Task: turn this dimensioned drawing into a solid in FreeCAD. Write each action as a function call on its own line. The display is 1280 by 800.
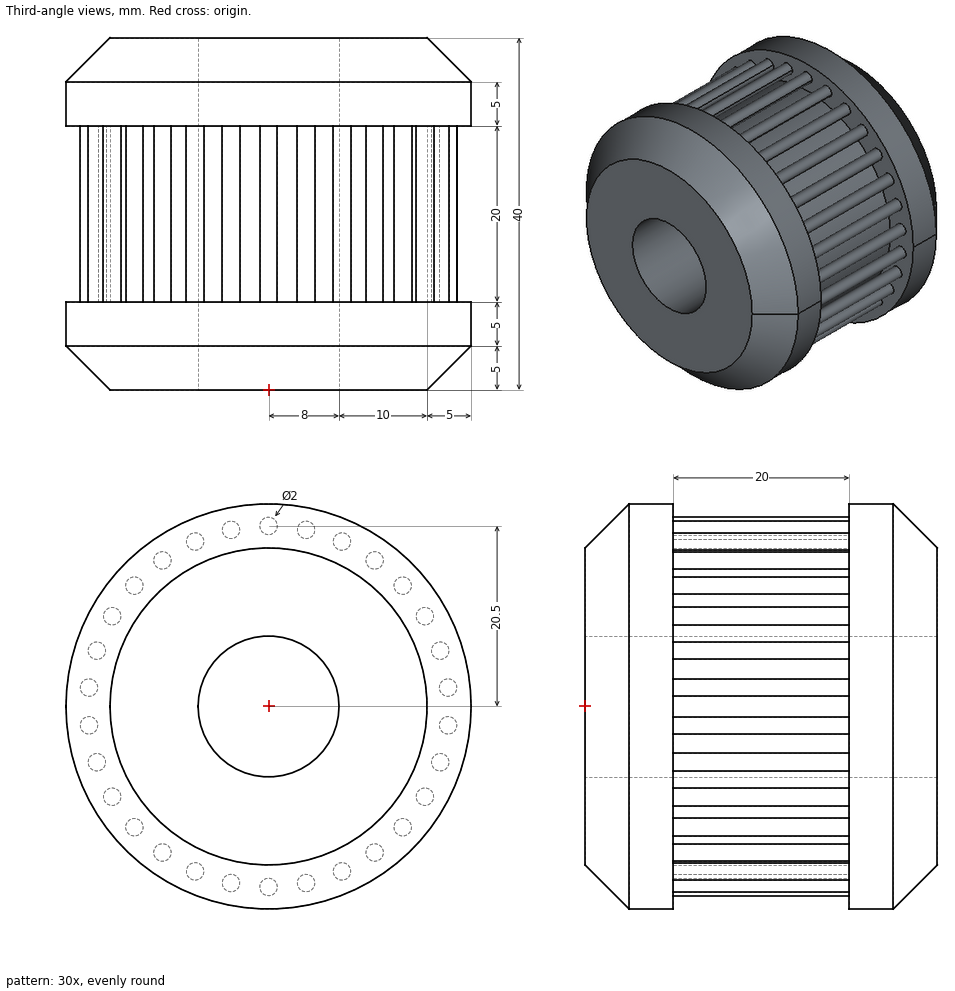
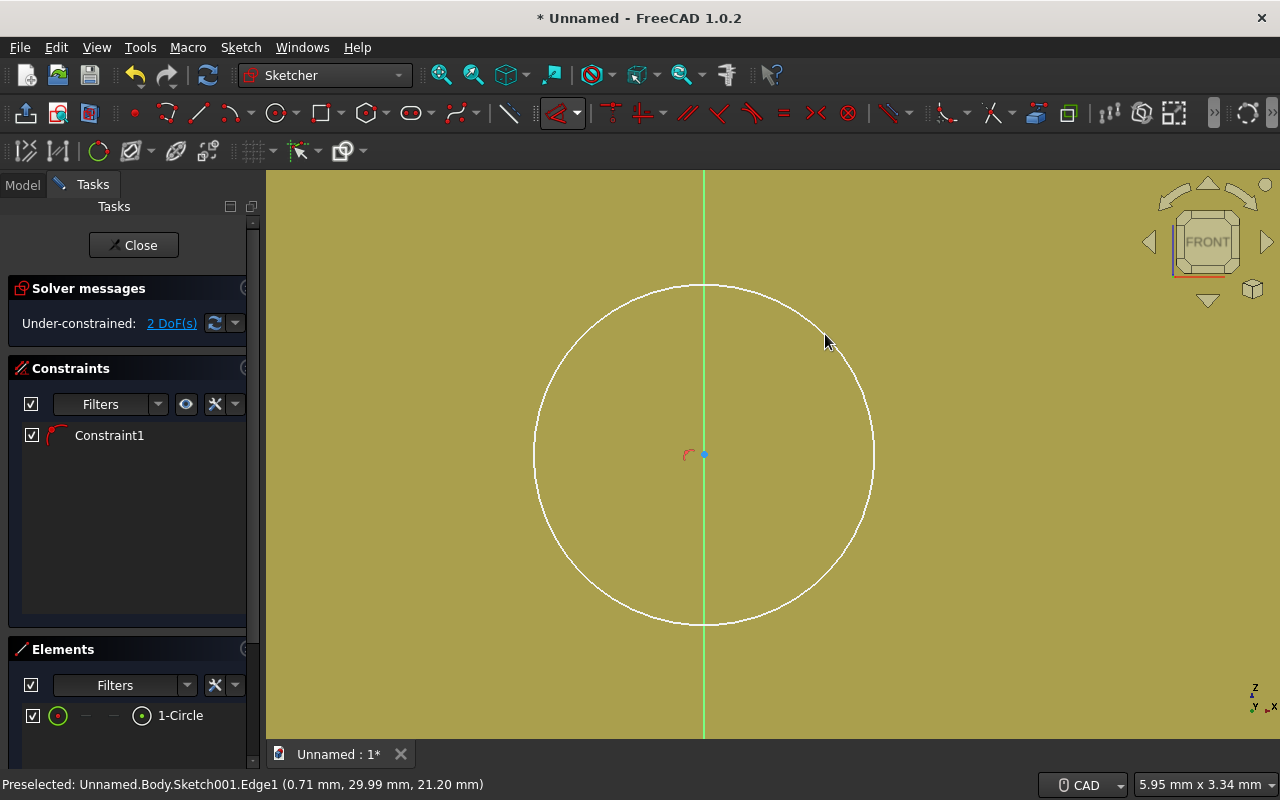
click(824, 334)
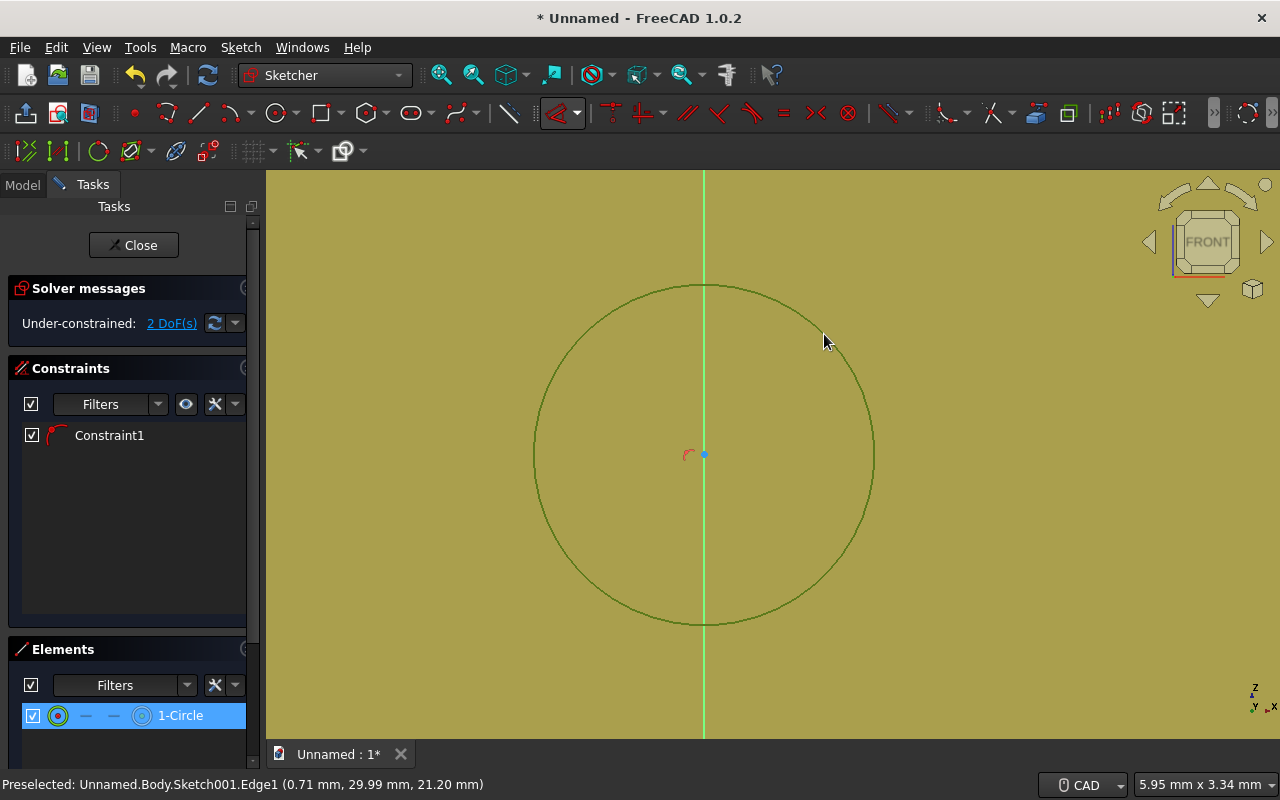
click(580, 114)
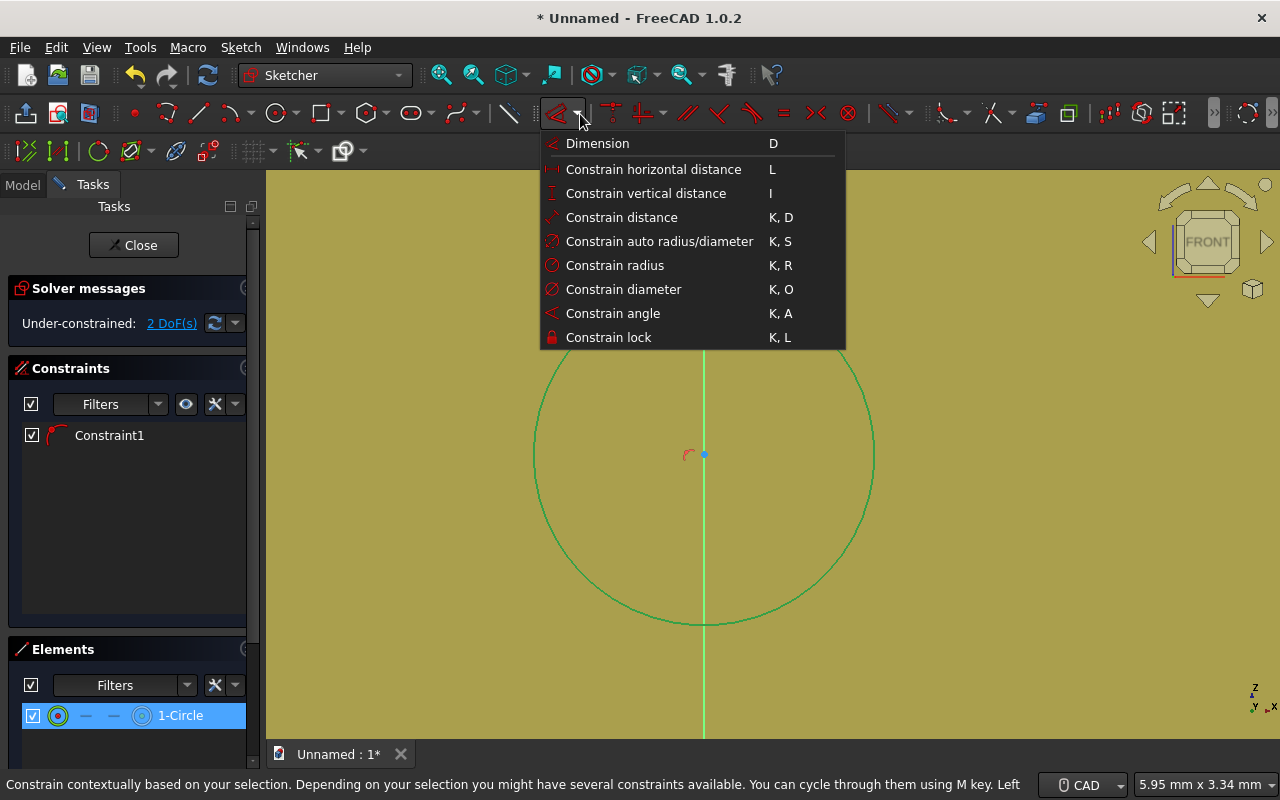
click(693, 289)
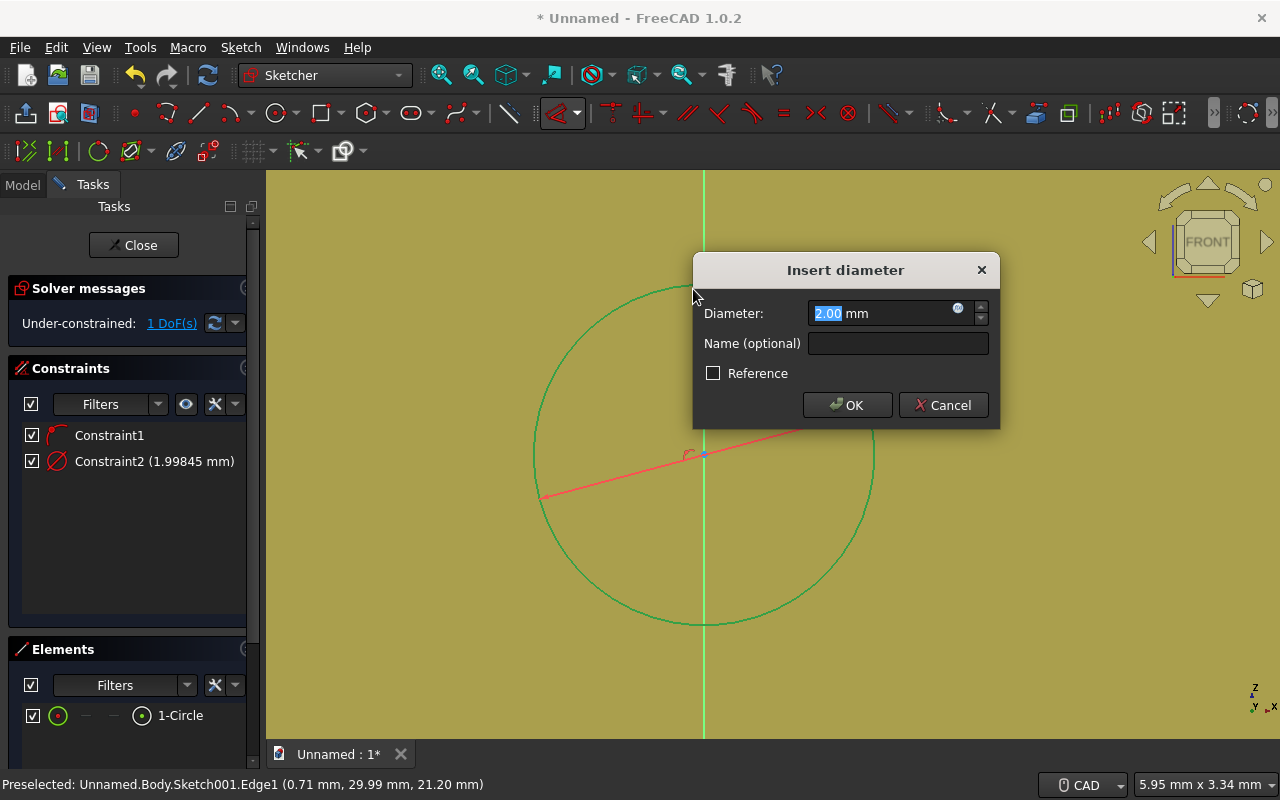
text(2)
key(Return)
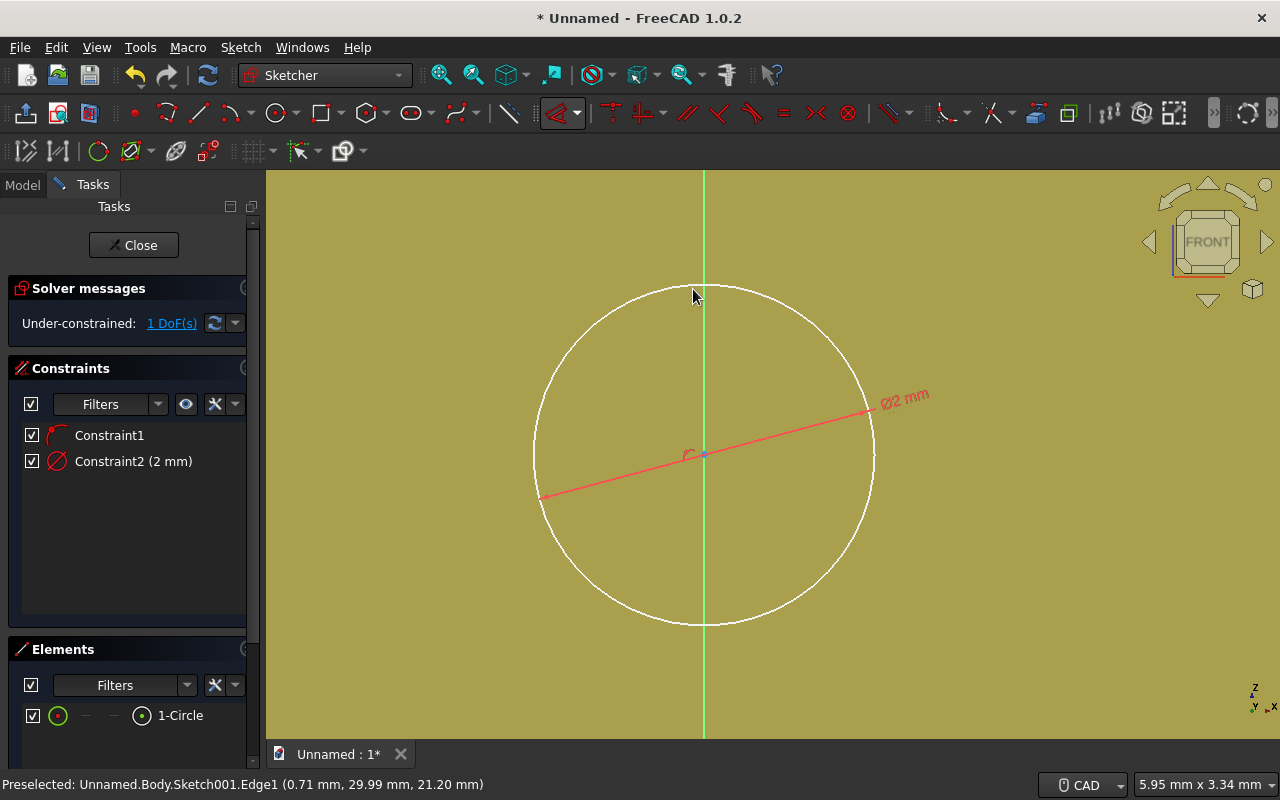
click(704, 455)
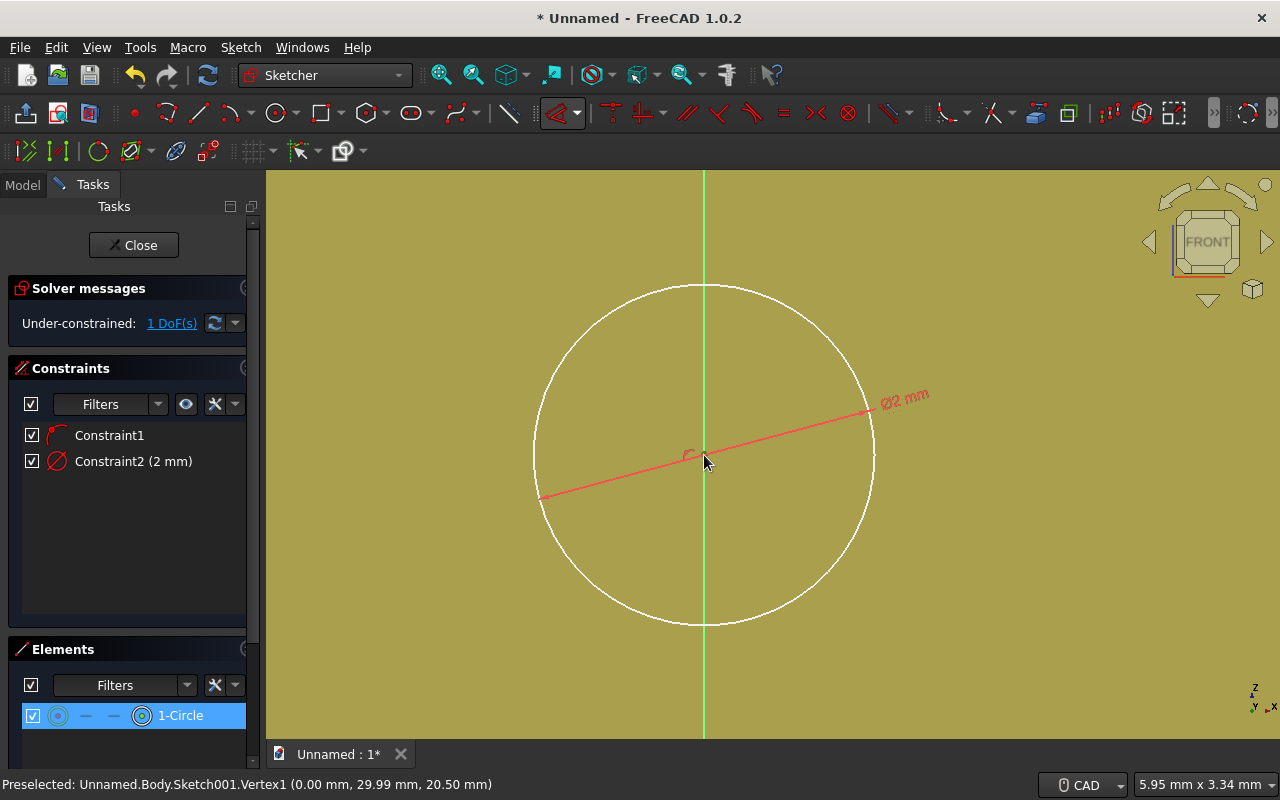
key(i)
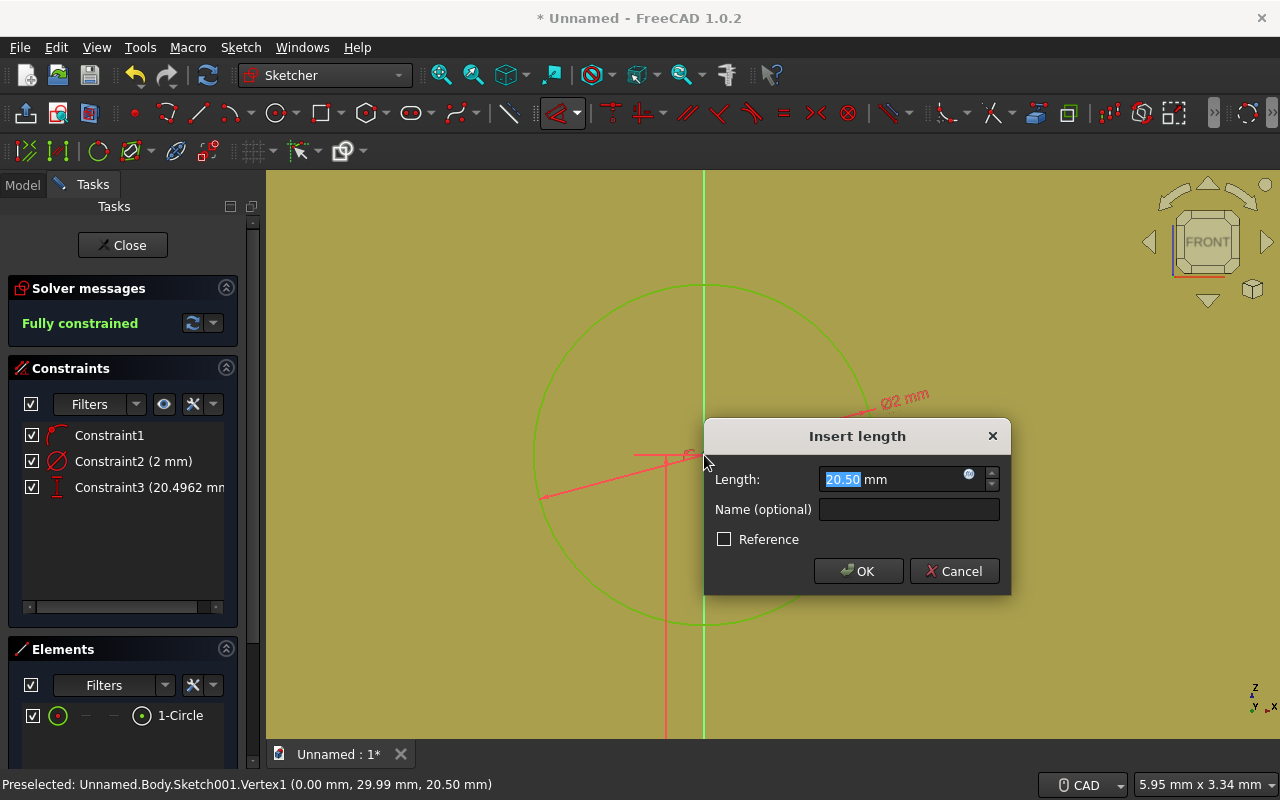
text(20.5)
key(Return)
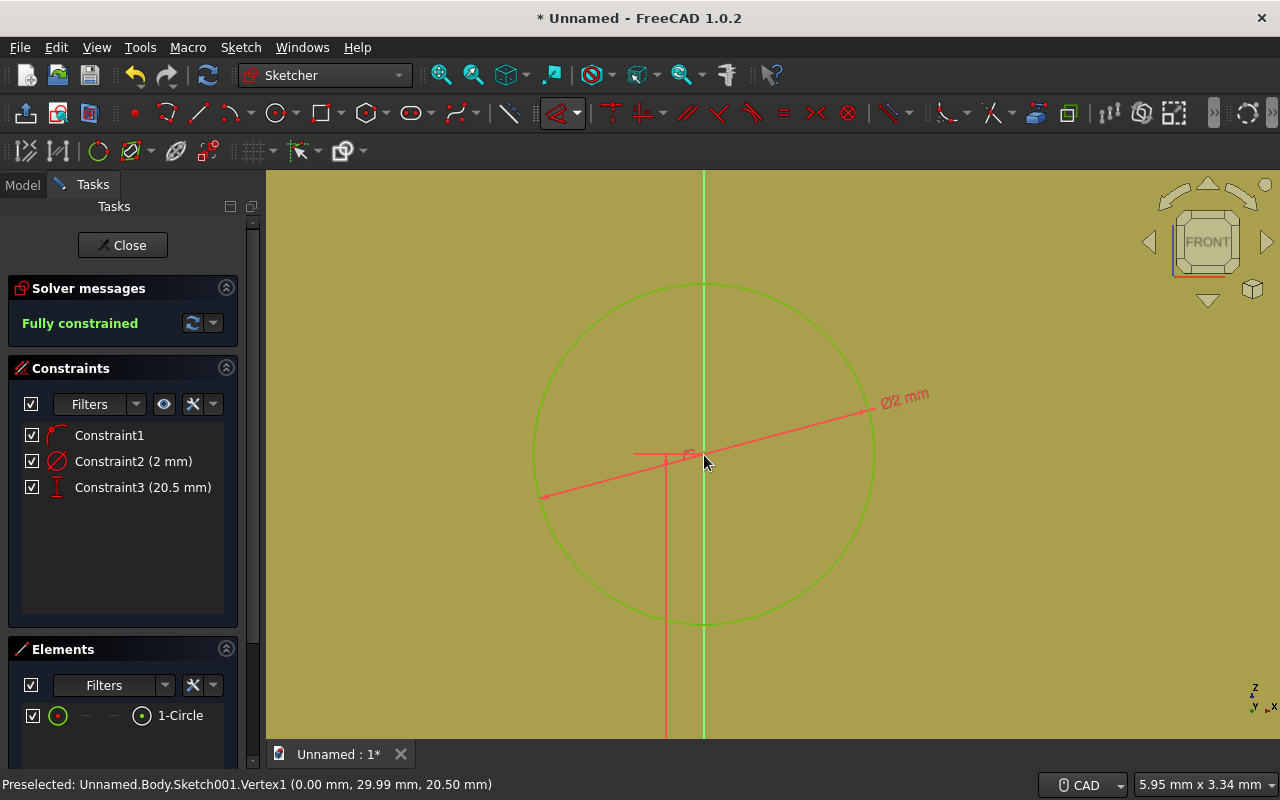
click(123, 245)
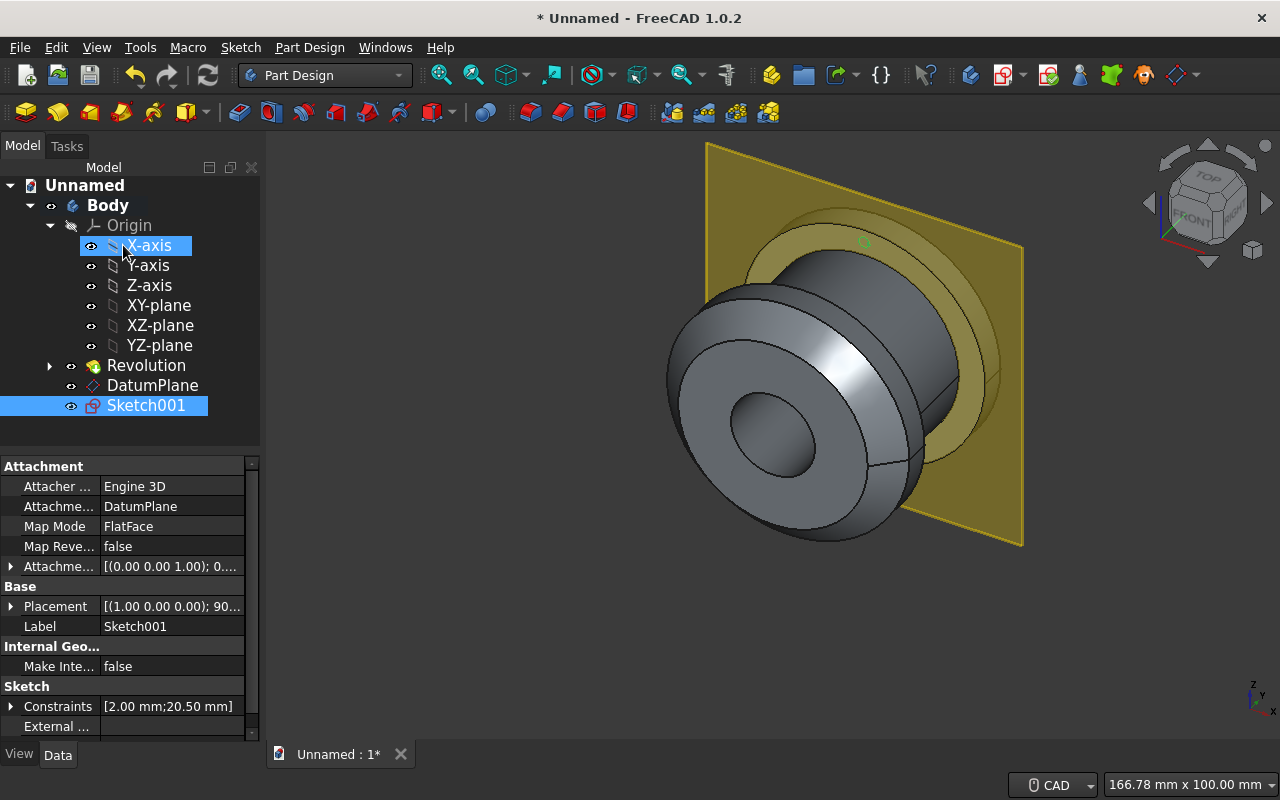
click(26, 112)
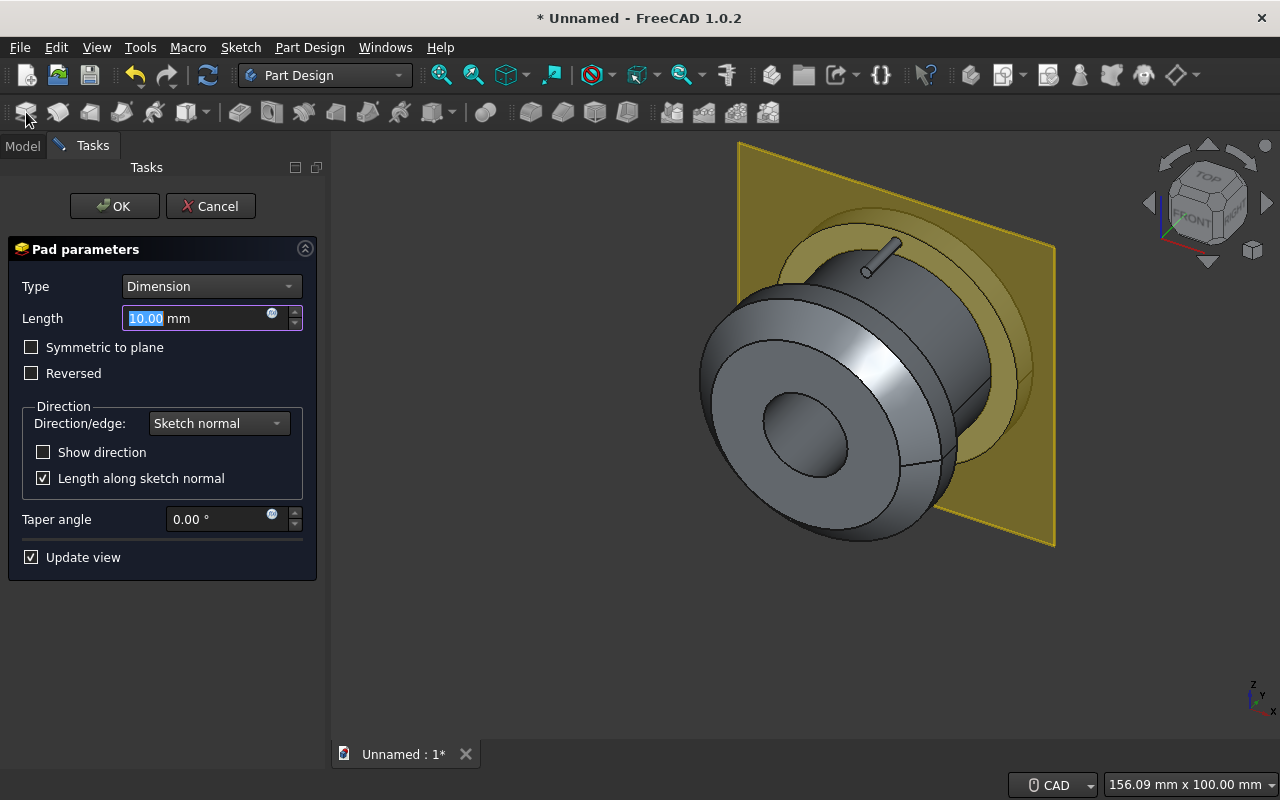
text(20)
key(Tab)